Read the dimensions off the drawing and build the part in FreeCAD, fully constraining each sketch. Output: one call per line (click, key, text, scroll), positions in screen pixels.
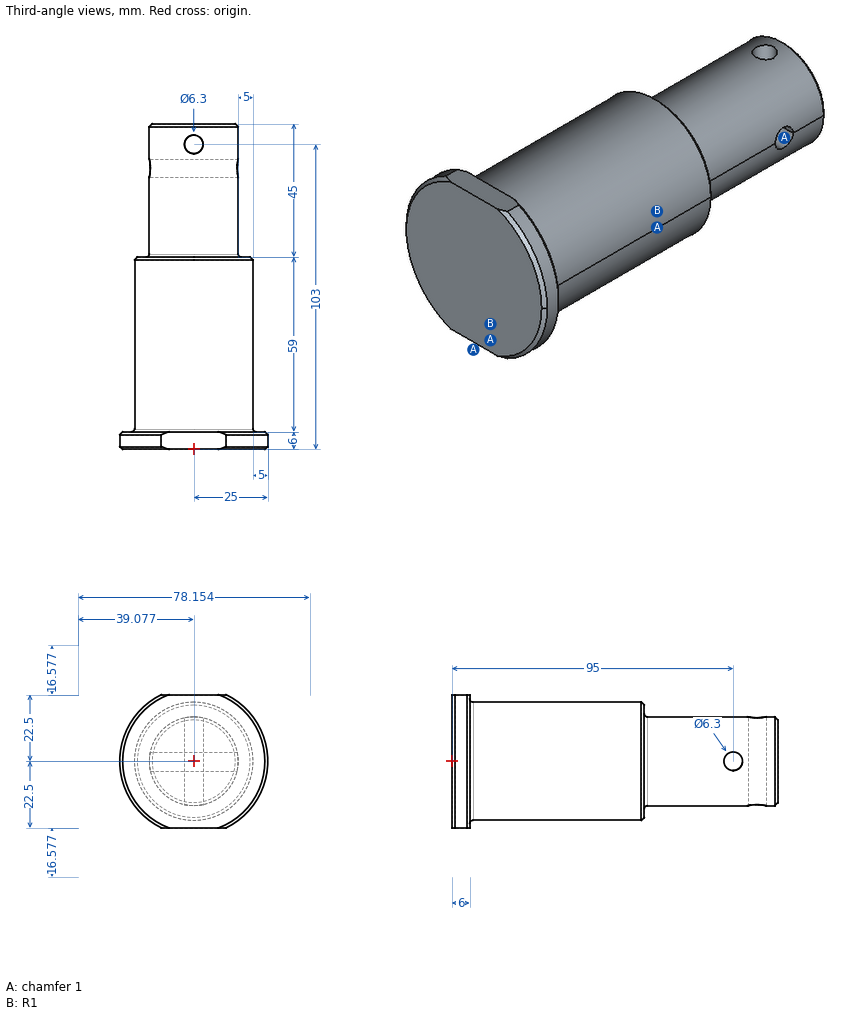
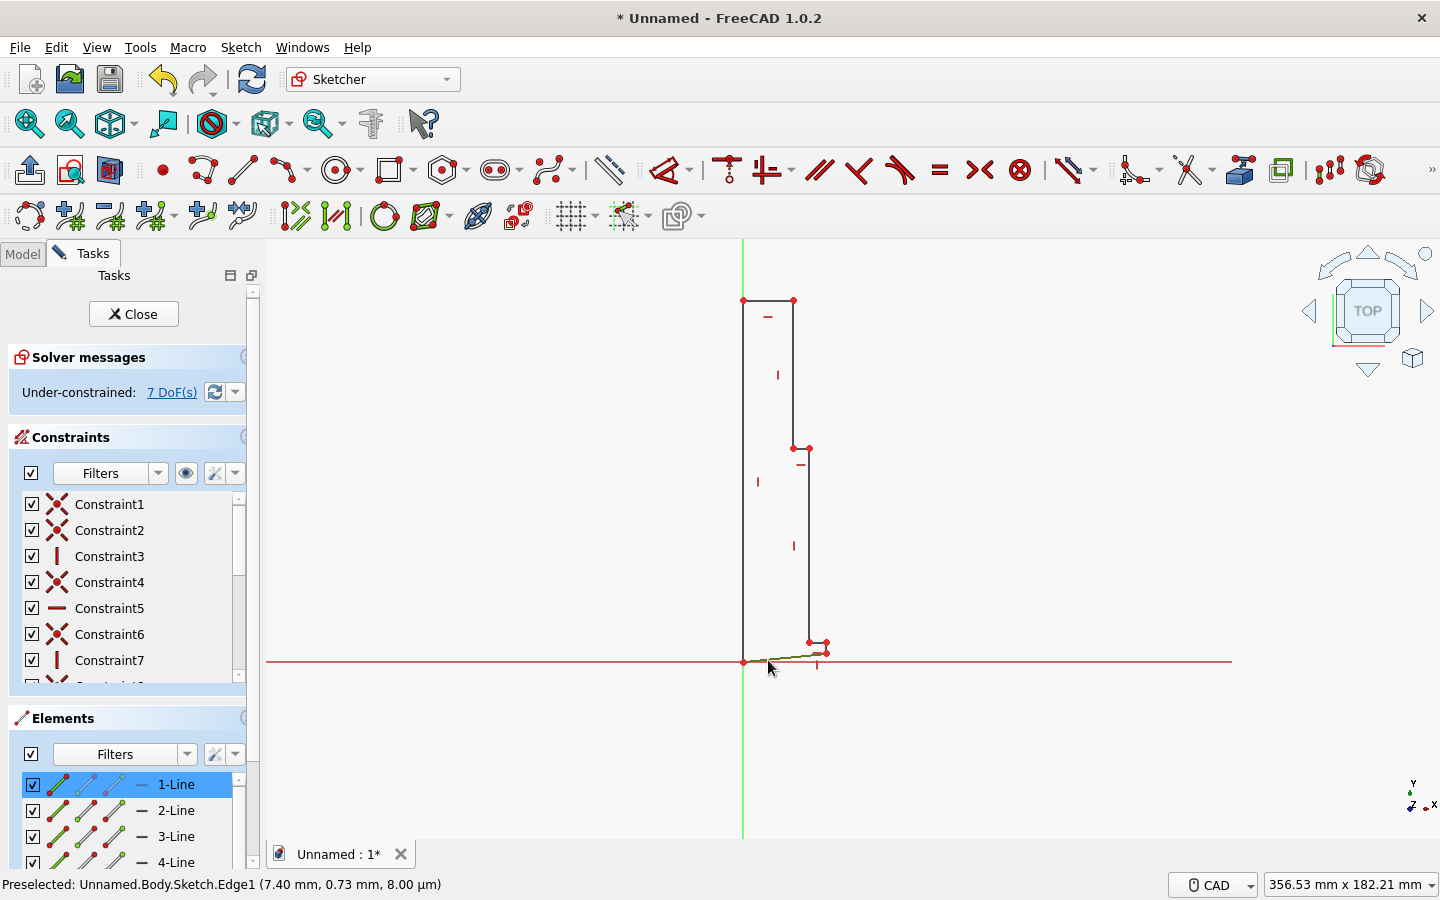
key(h)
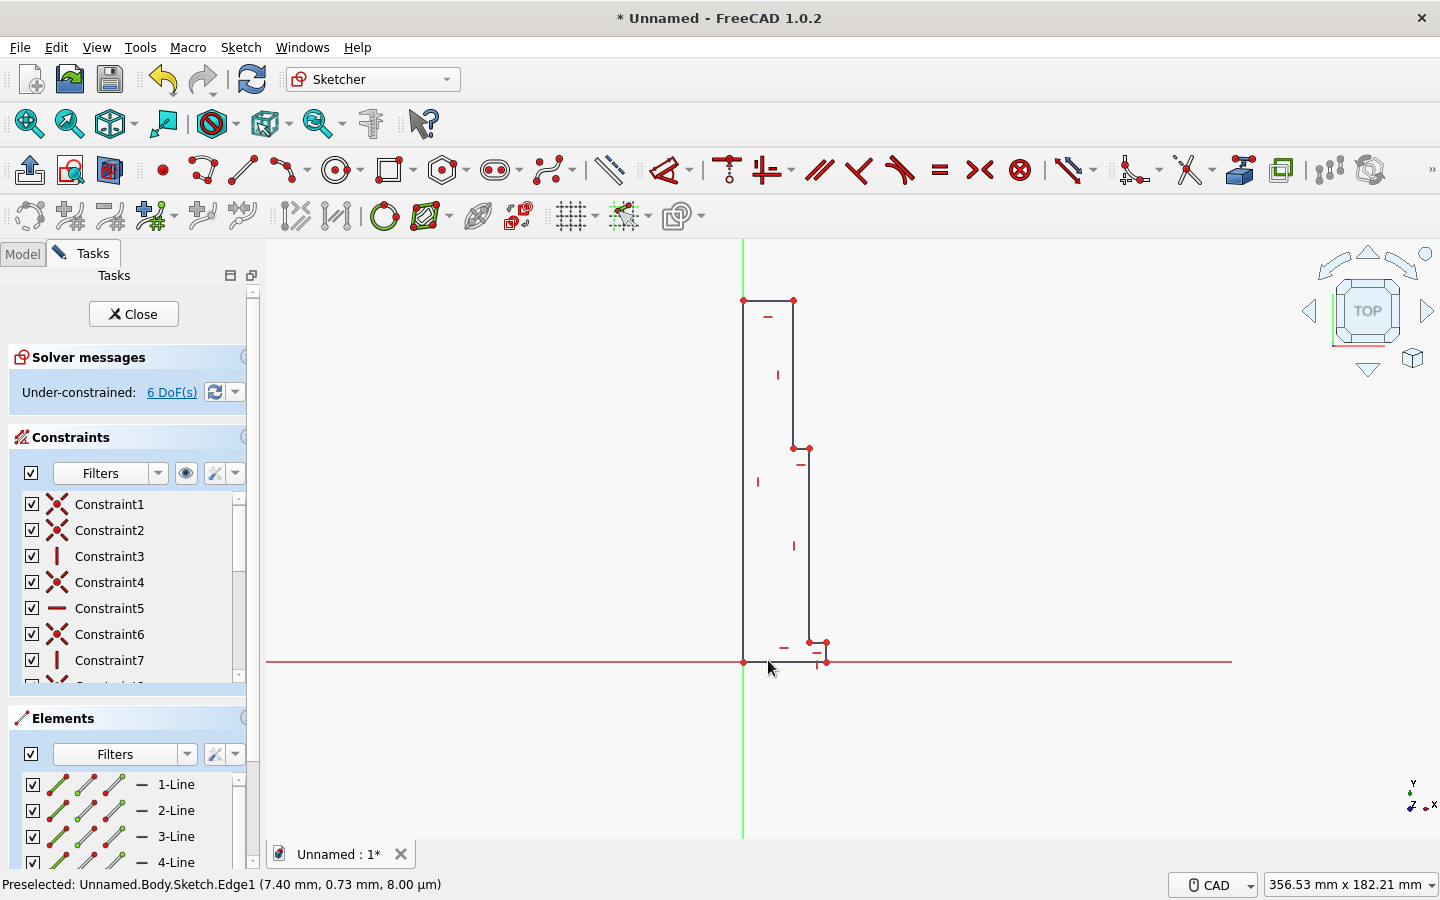
key(d)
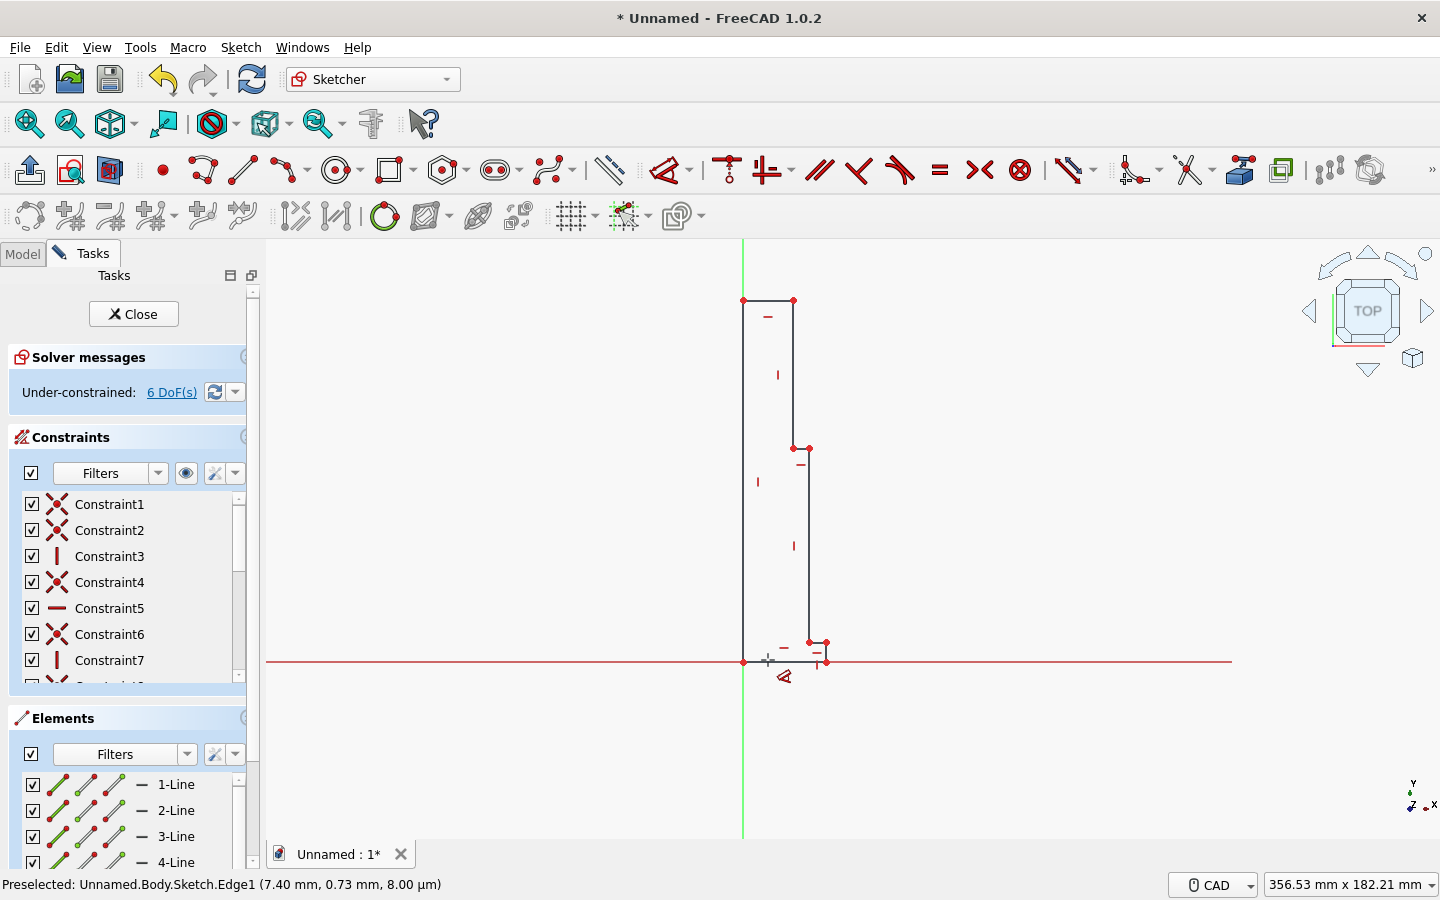
scroll(826, 653, up, 4)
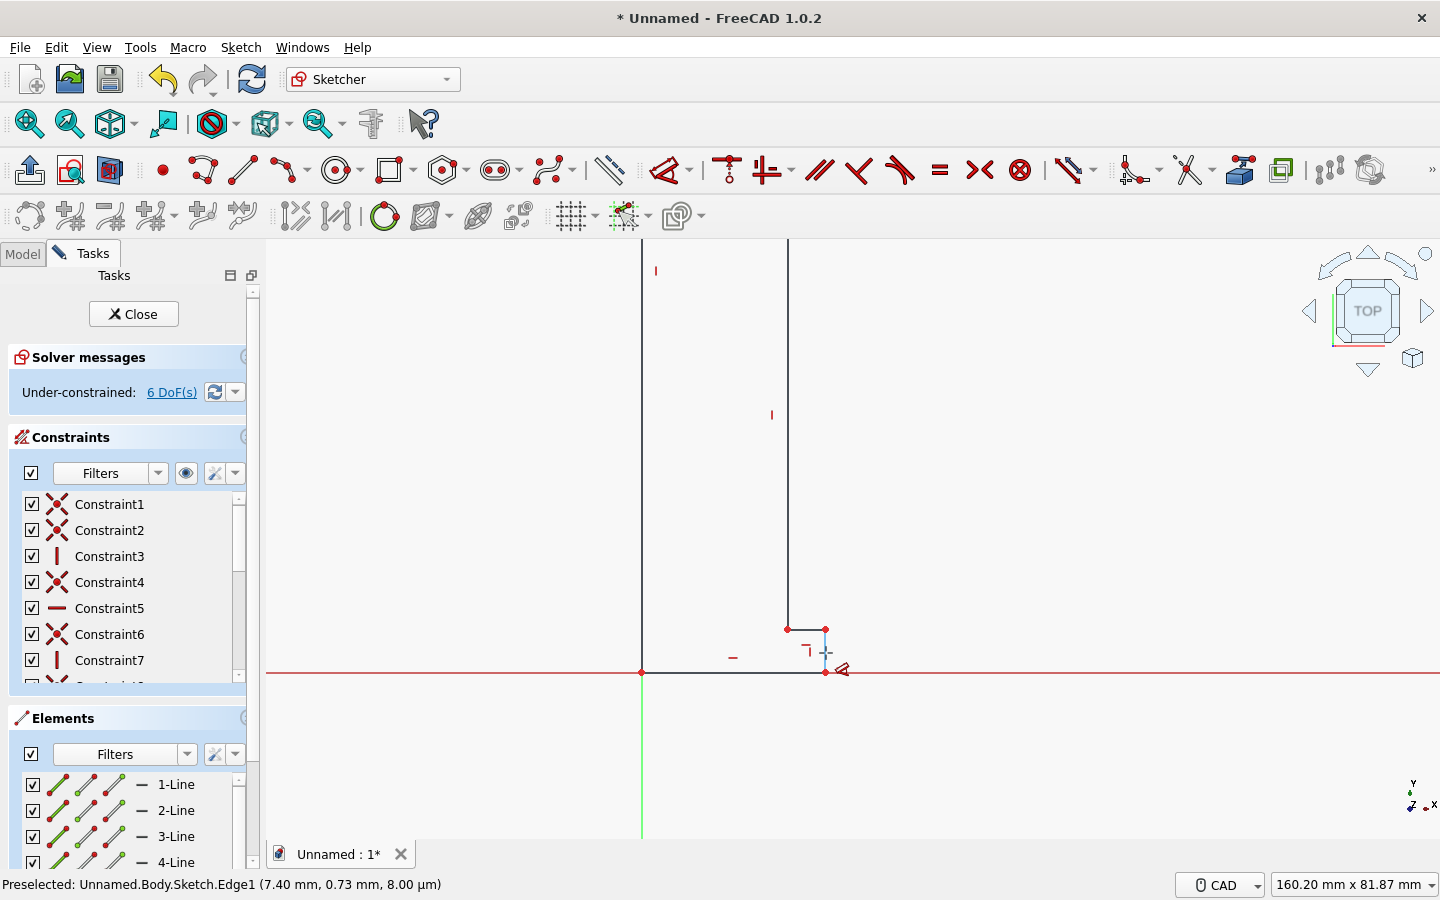
click(825, 651)
click(859, 651)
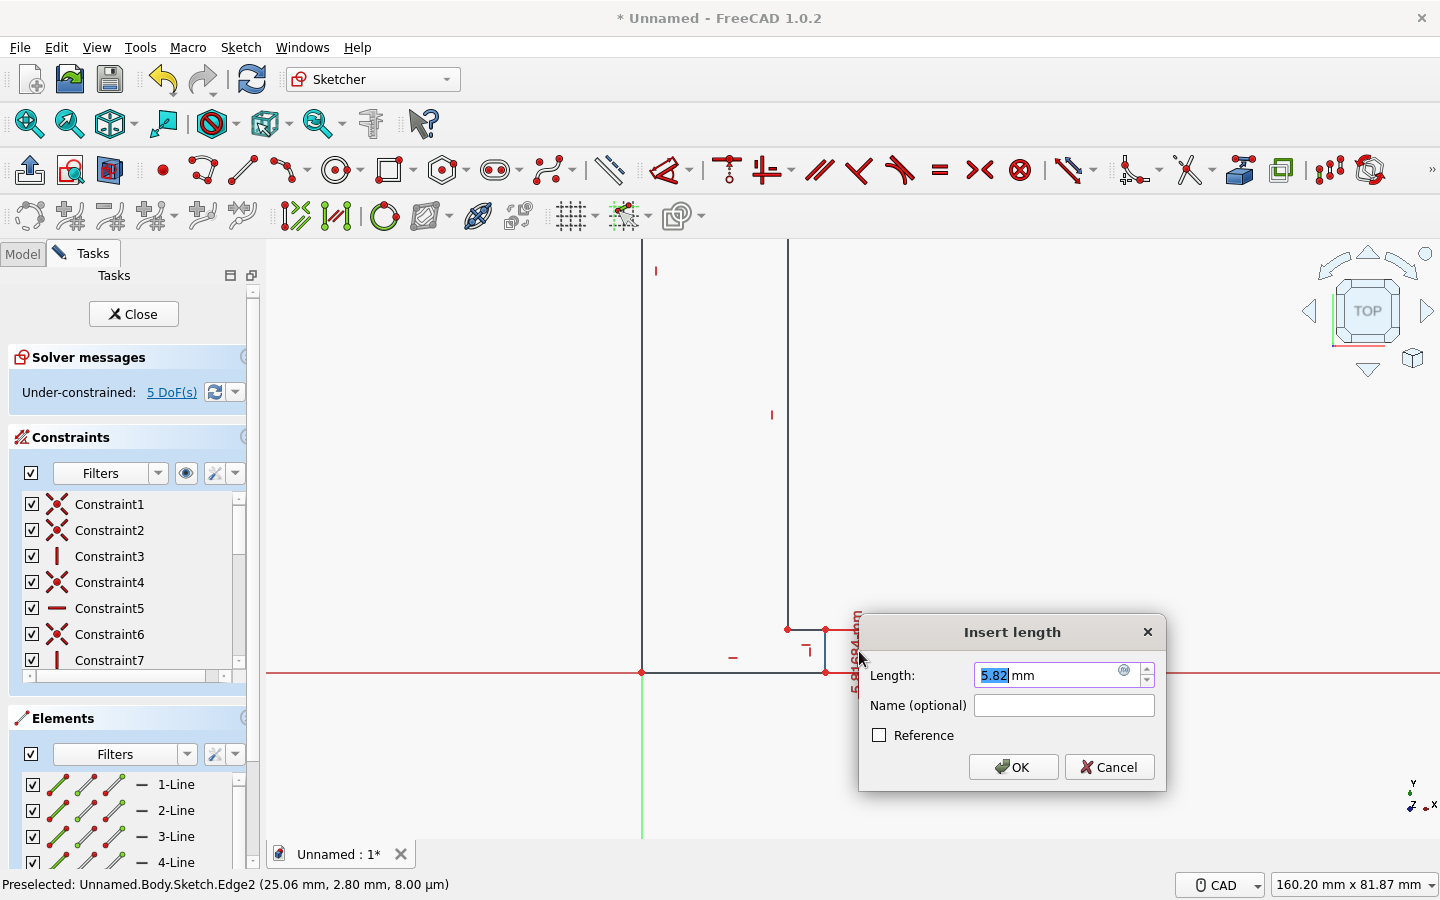
text(6)
key(Return)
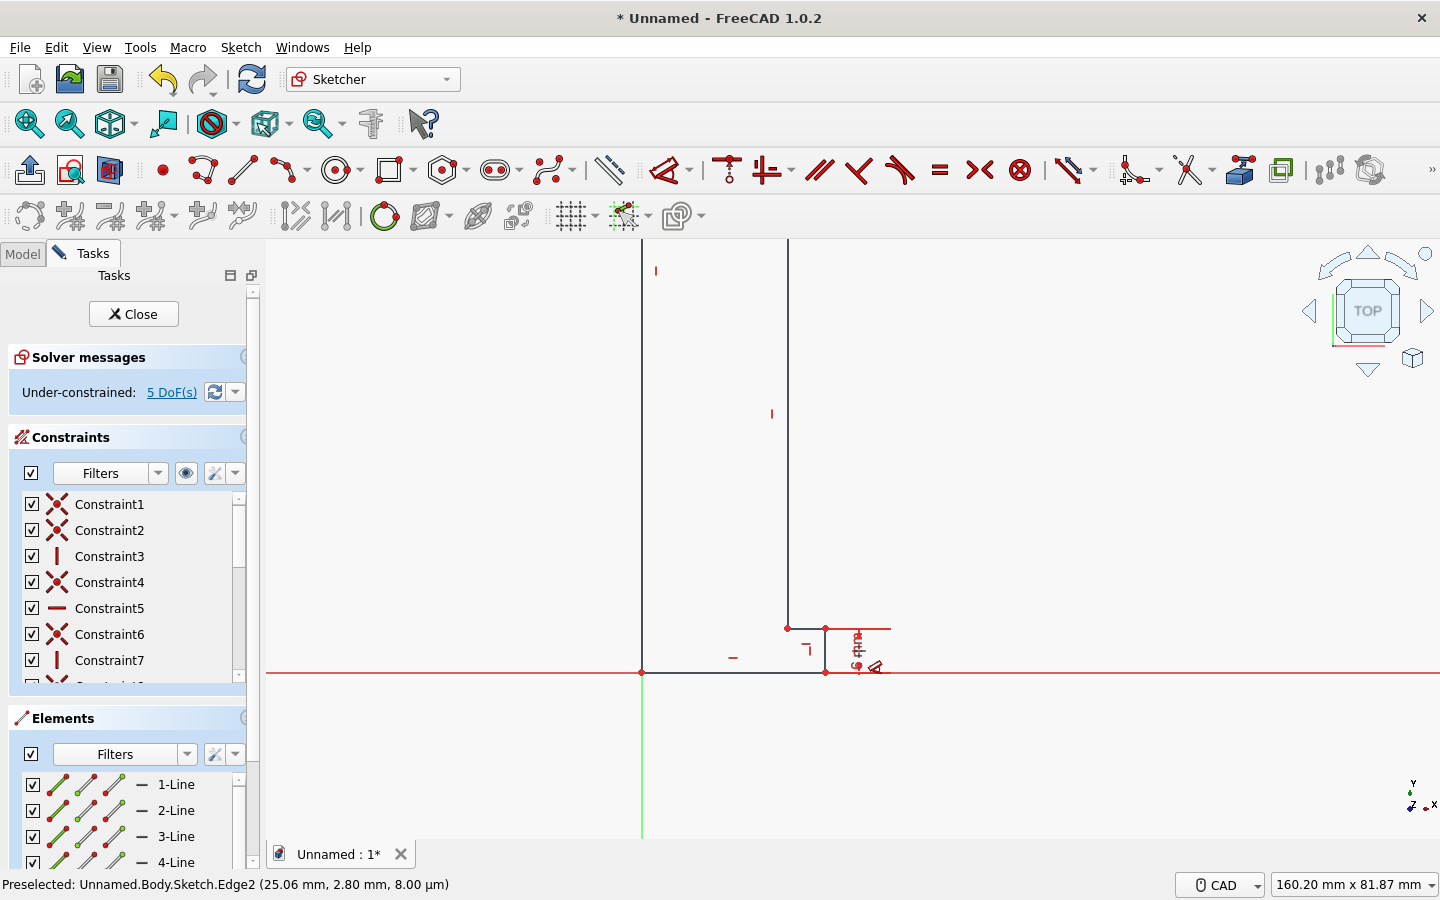
click(814, 629)
click(806, 595)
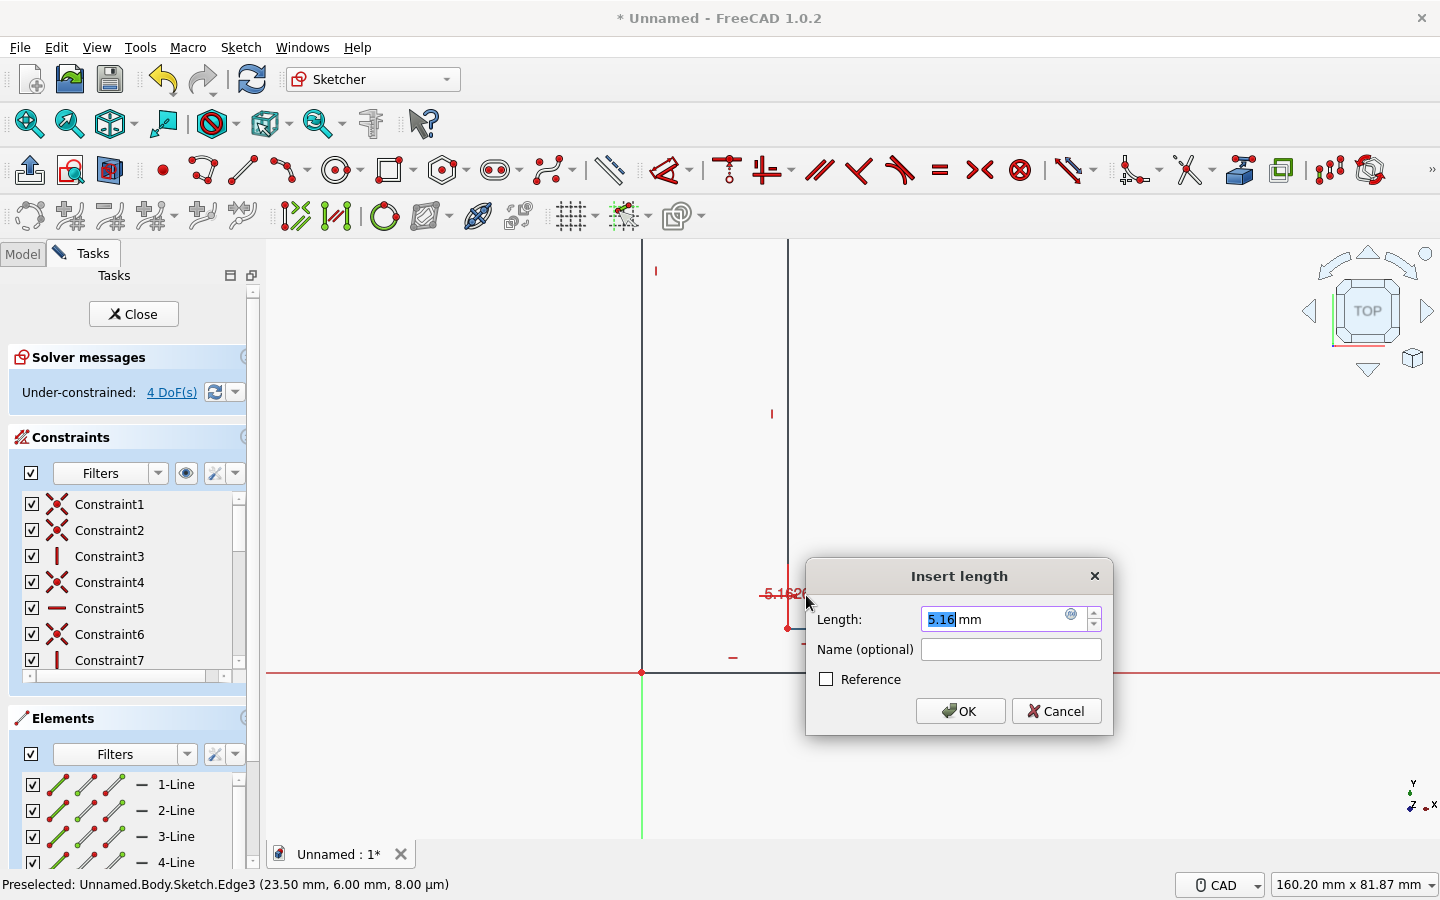
text(5)
key(Return)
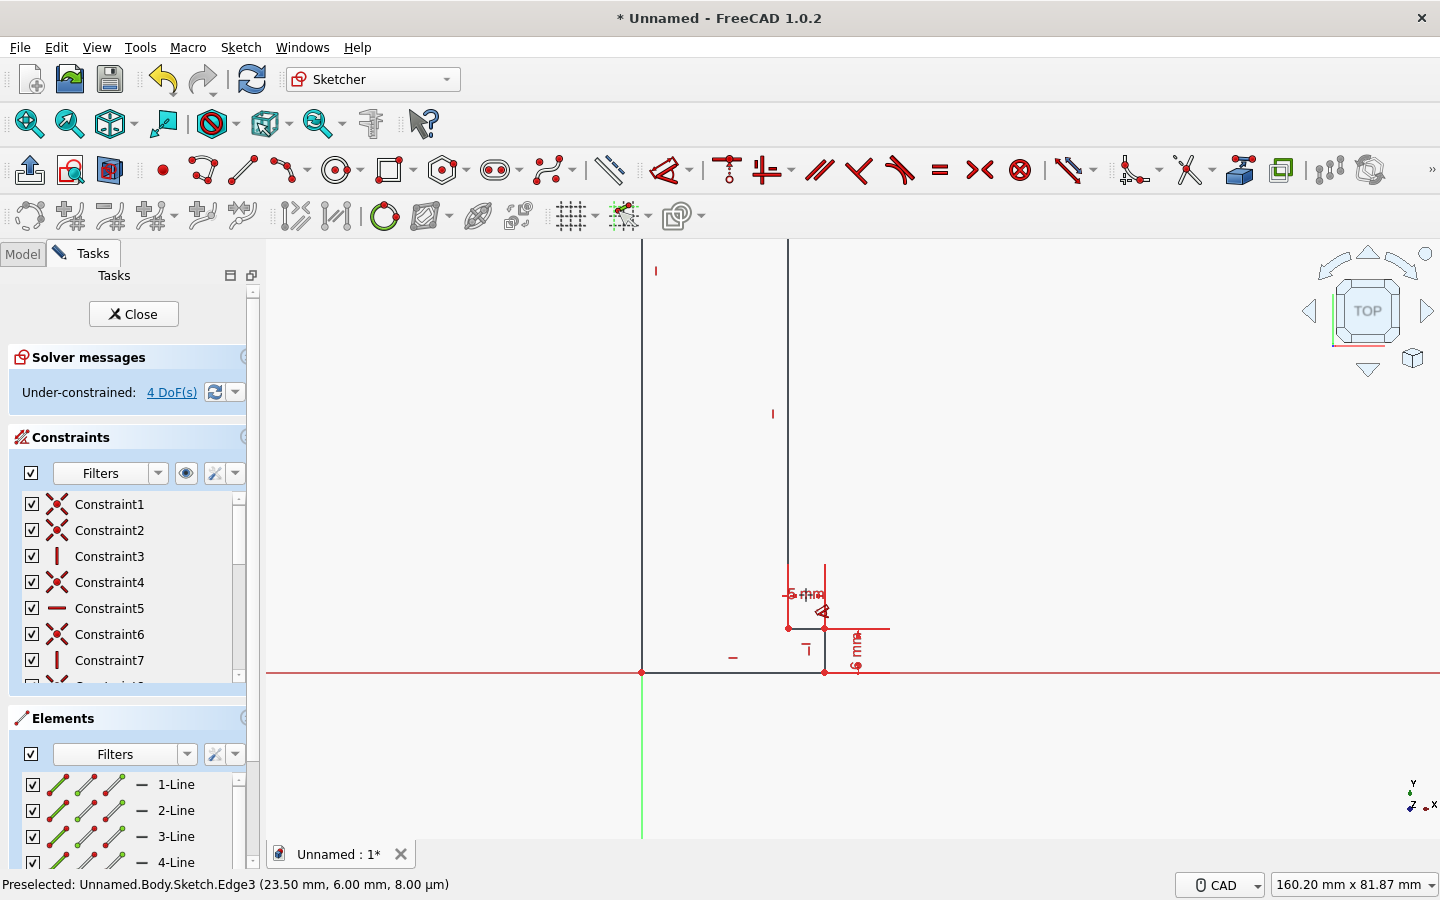
scroll(826, 759, down, 4)